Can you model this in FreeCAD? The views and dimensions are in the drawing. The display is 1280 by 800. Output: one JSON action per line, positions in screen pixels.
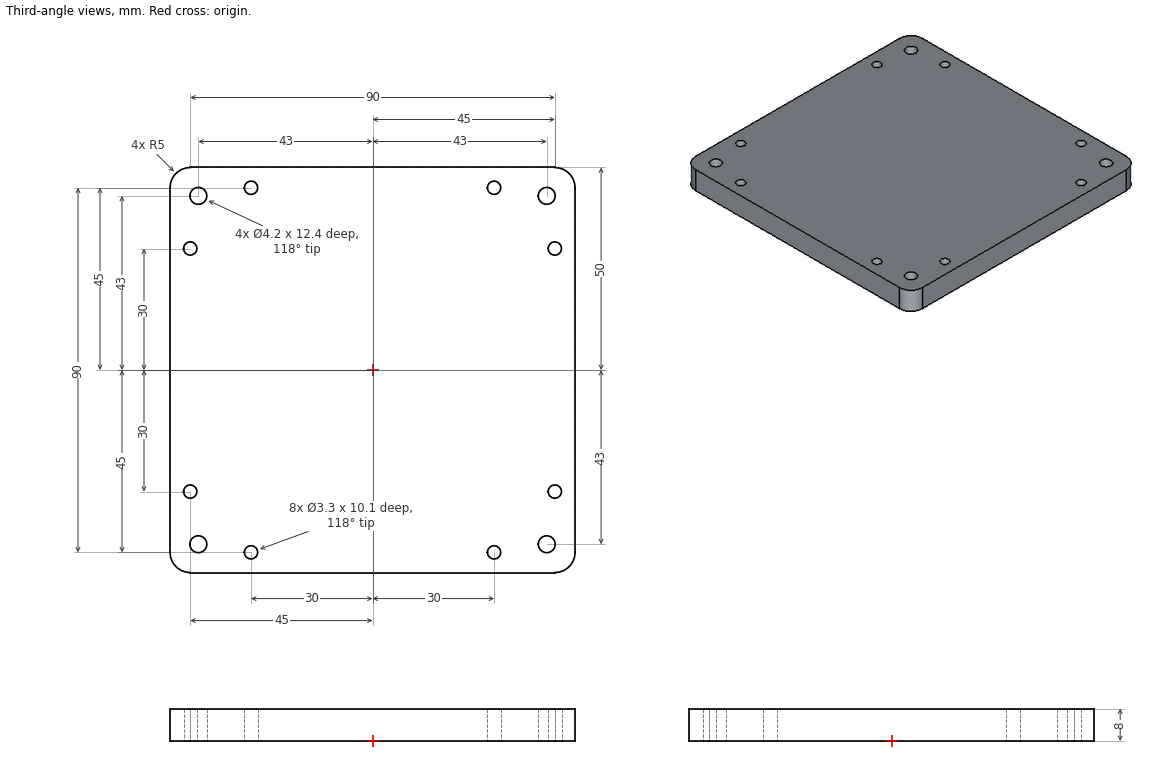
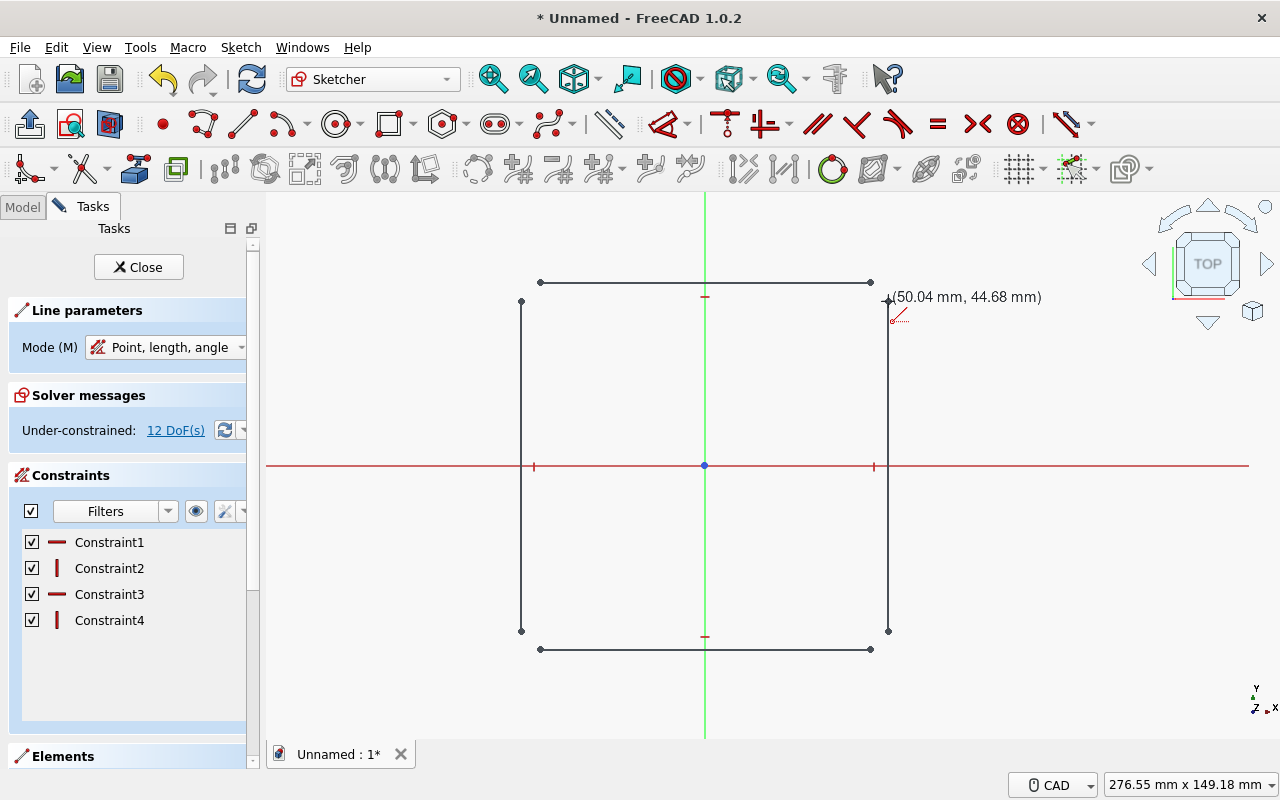
{"action": "key", "text": "g 3 a"}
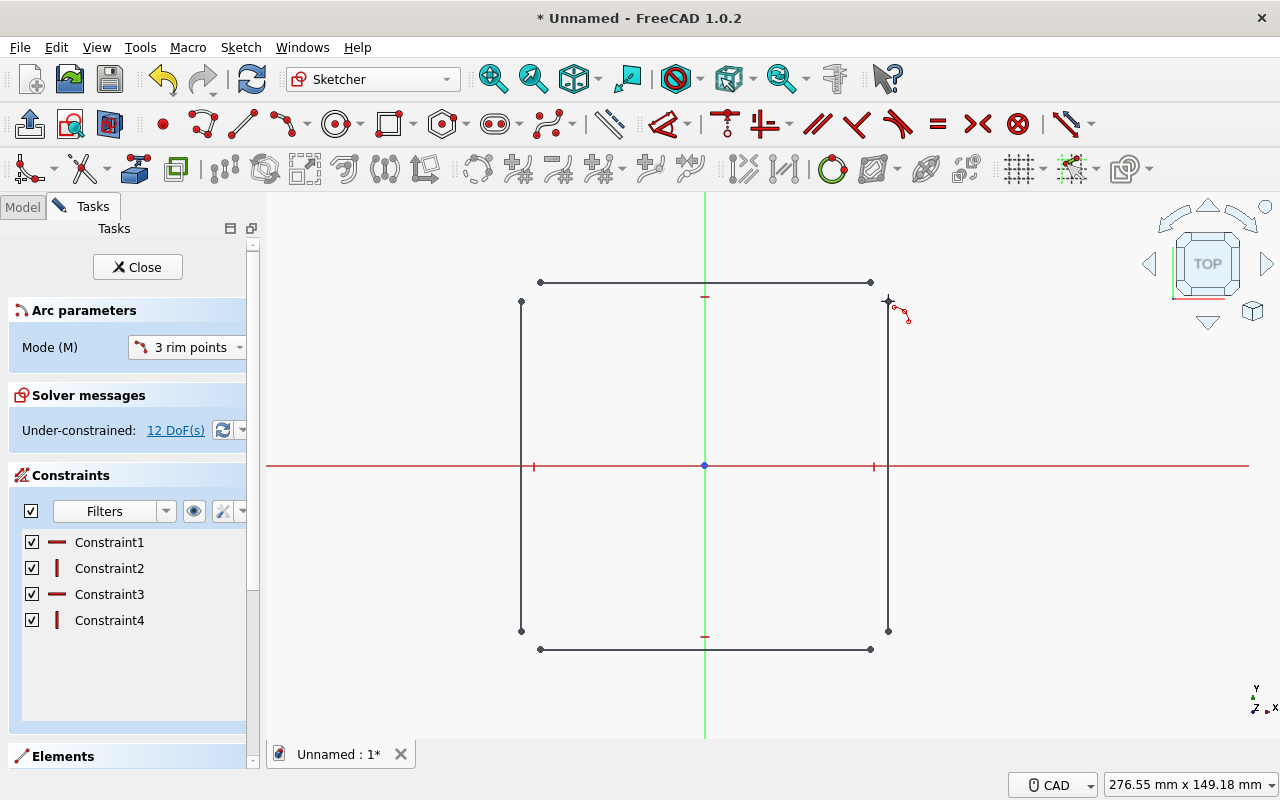
{"action": "left_click", "coordinate": [540, 283]}
{"action": "left_click", "coordinate": [521, 302]}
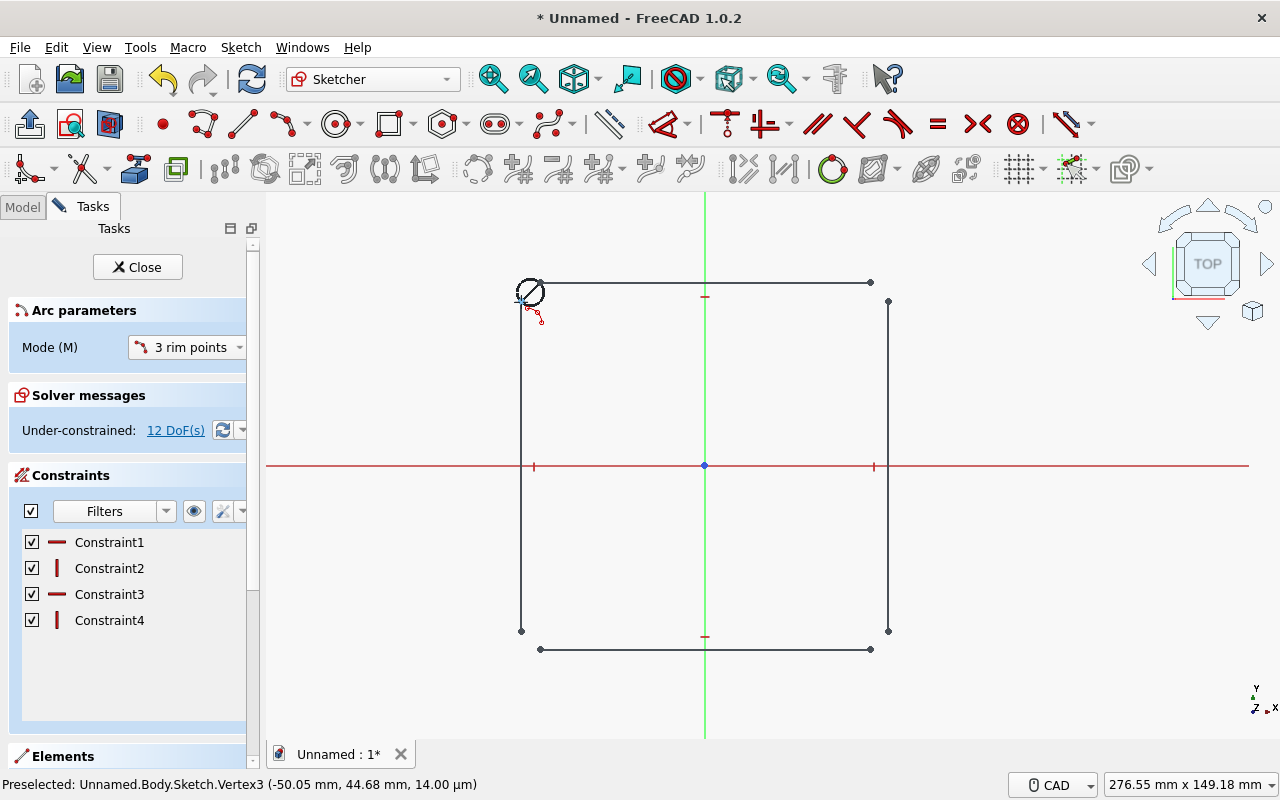
{"action": "scroll", "coordinate": [527, 288], "scroll_direction": "up", "scroll_amount": 6}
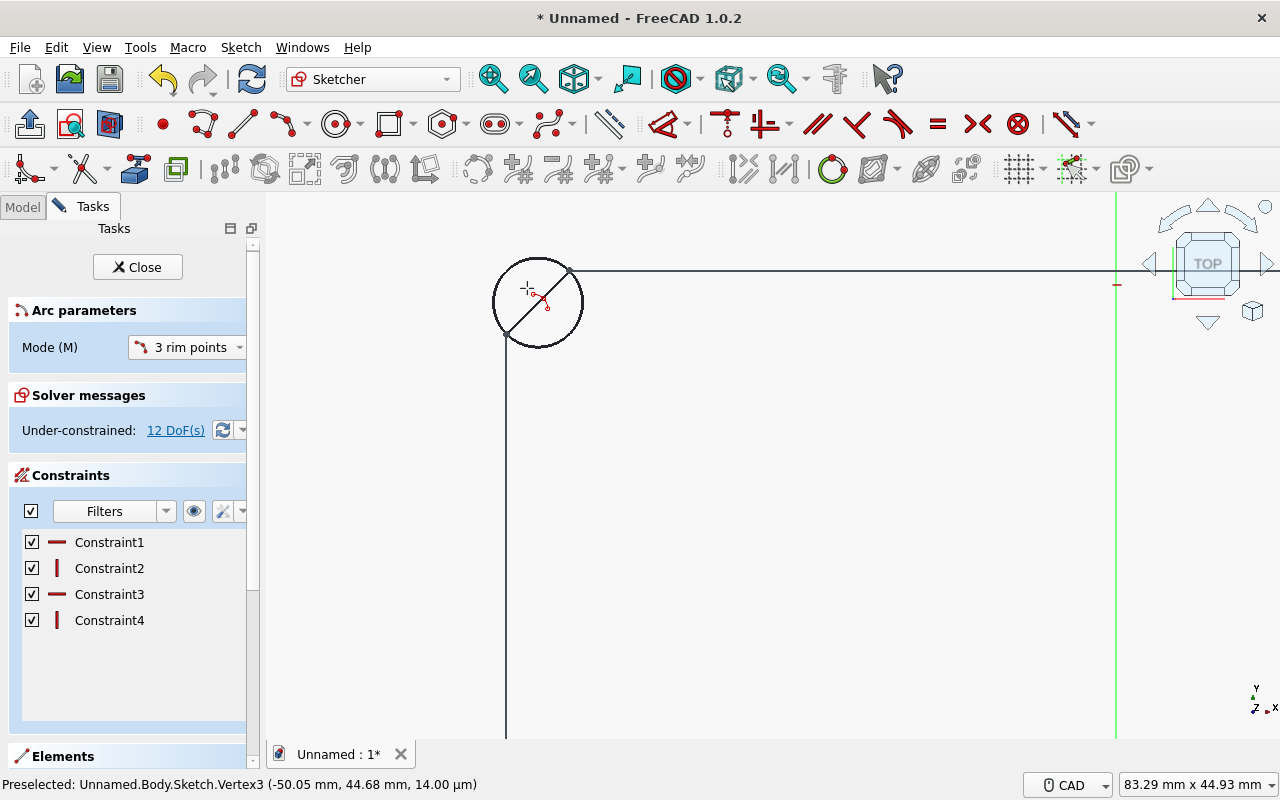
{"action": "left_click", "coordinate": [525, 287]}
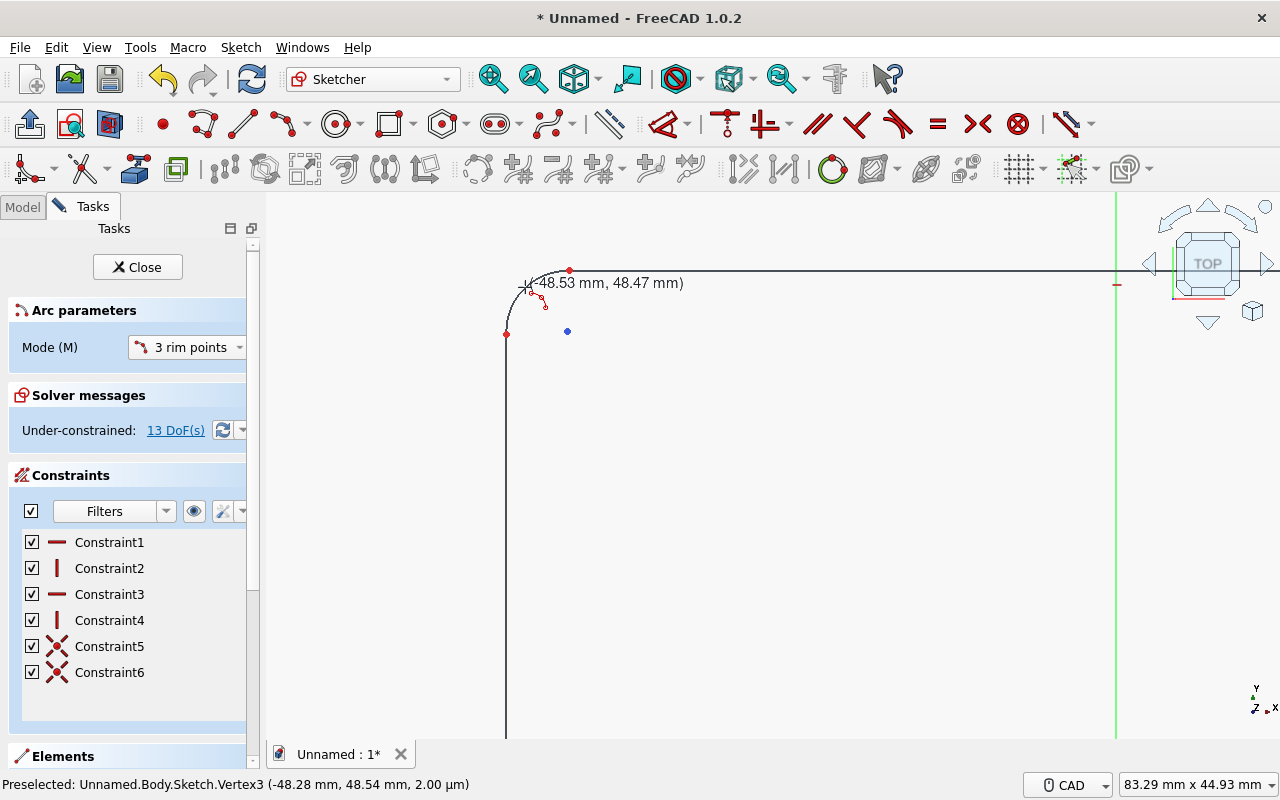
{"action": "scroll", "coordinate": [527, 288], "scroll_direction": "down", "scroll_amount": 6}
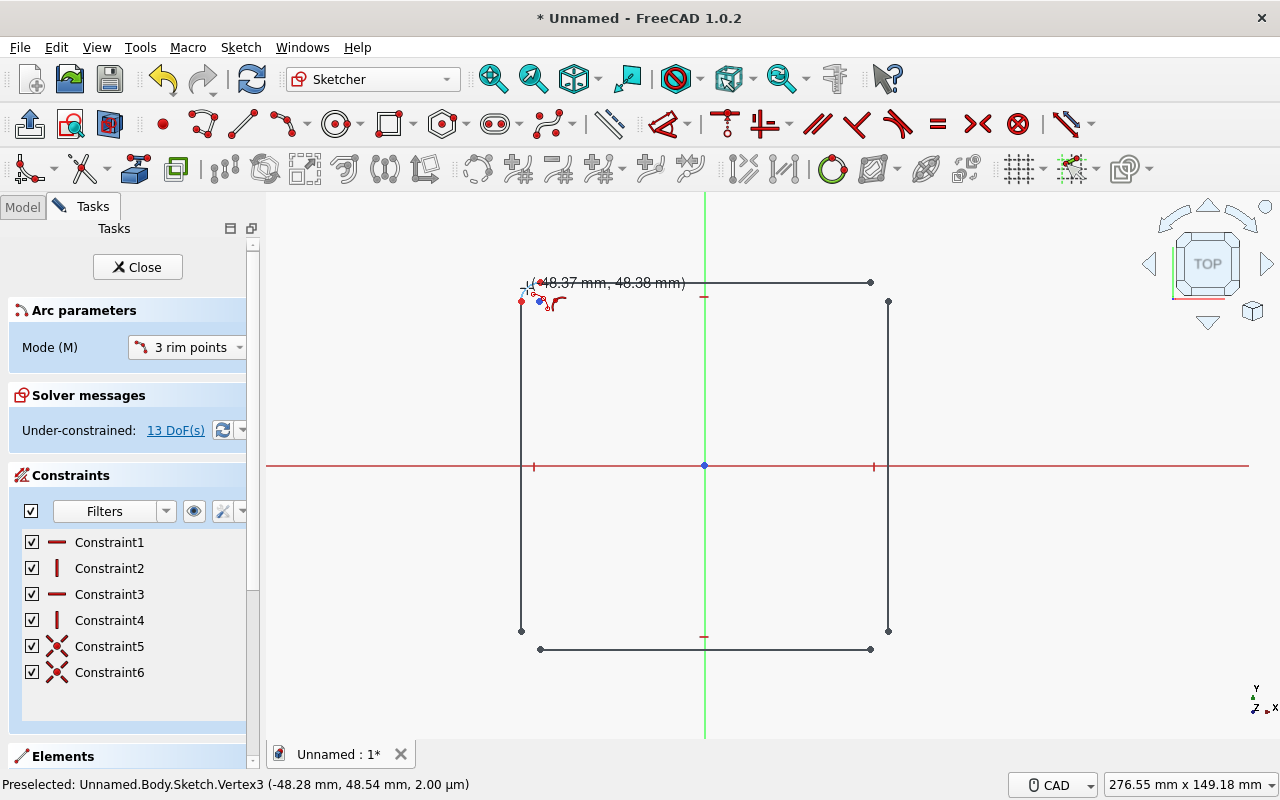
{"action": "left_click", "coordinate": [521, 632]}
{"action": "left_click", "coordinate": [540, 650]}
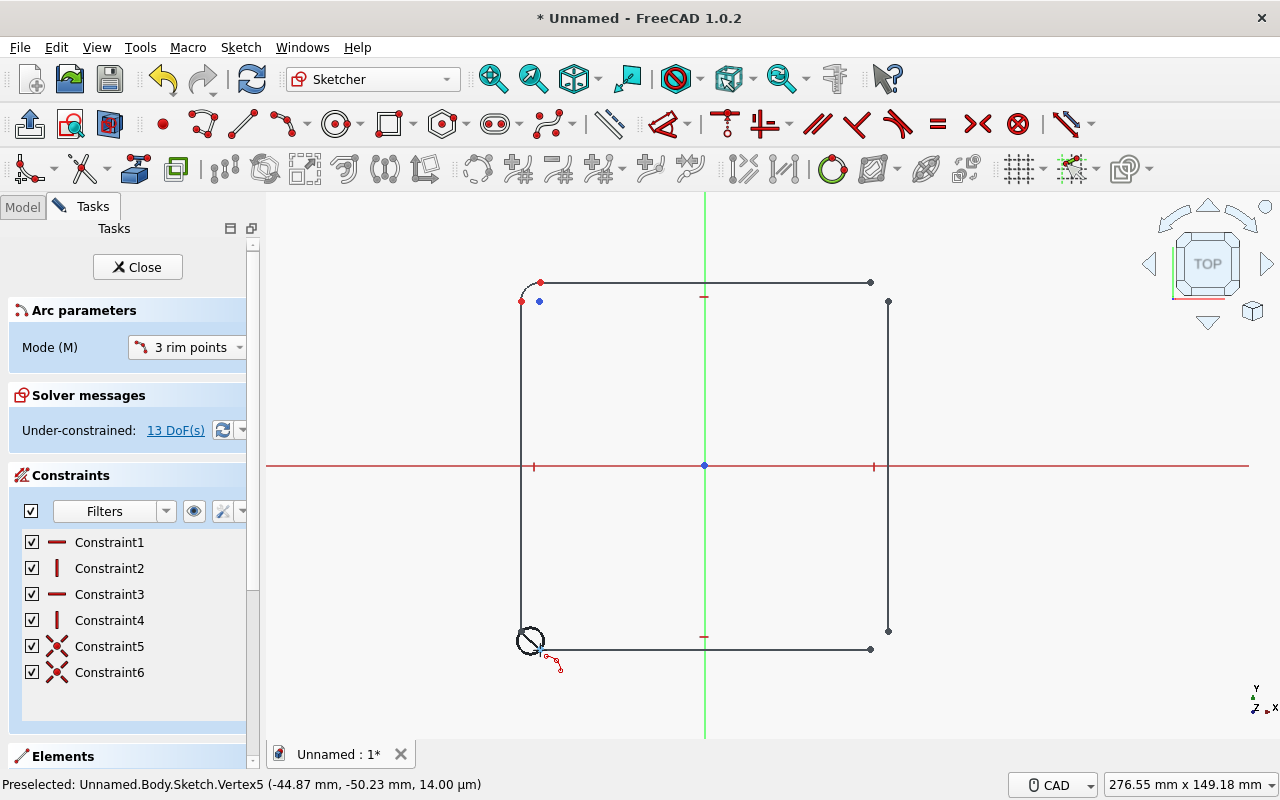
{"action": "scroll", "coordinate": [527, 644], "scroll_direction": "up", "scroll_amount": 6}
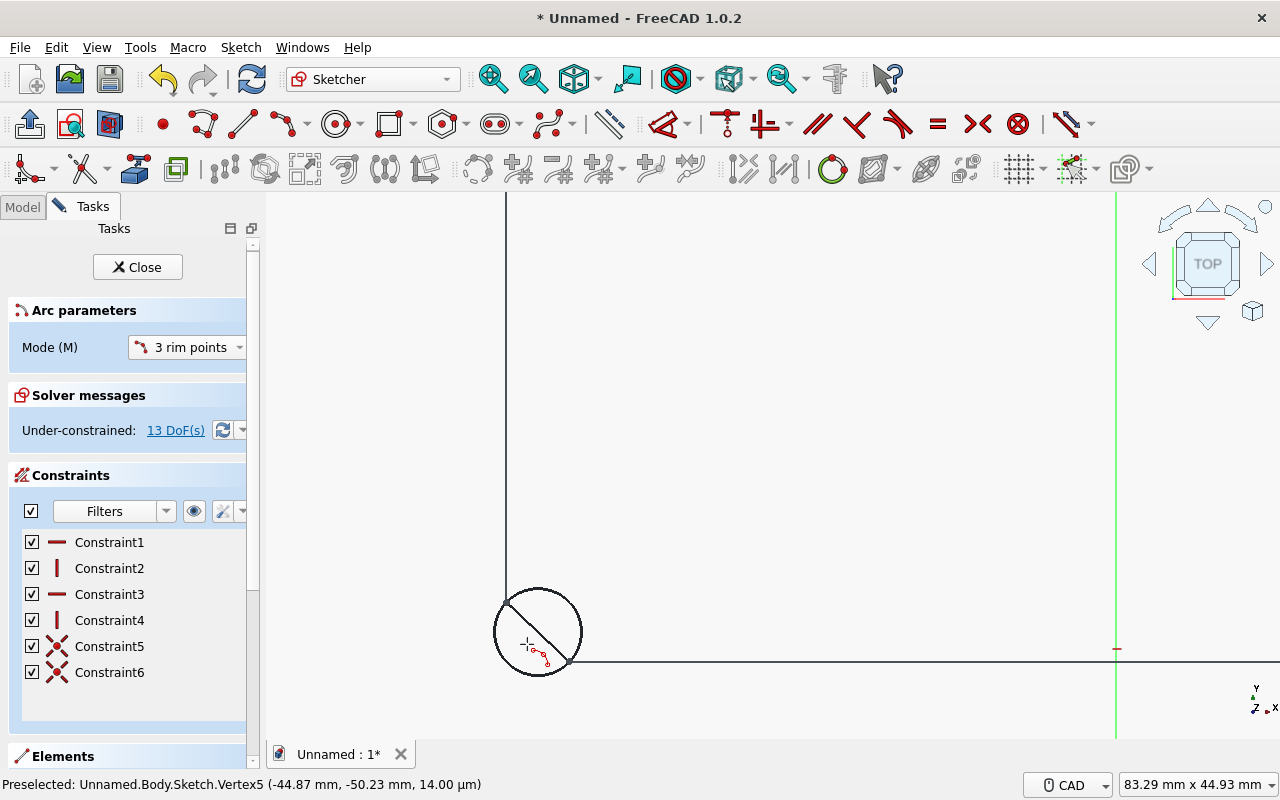
{"action": "left_click", "coordinate": [525, 641]}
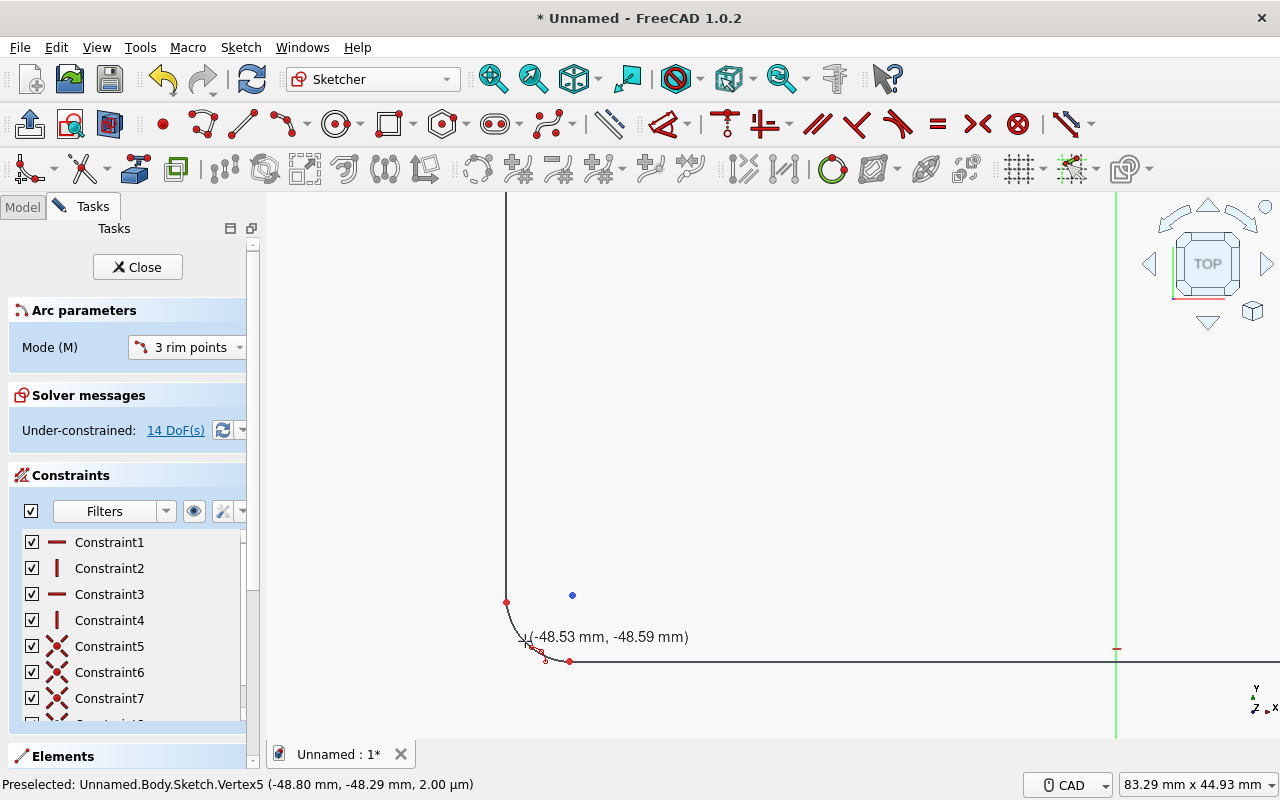
{"action": "scroll", "coordinate": [527, 644], "scroll_direction": "down", "scroll_amount": 6}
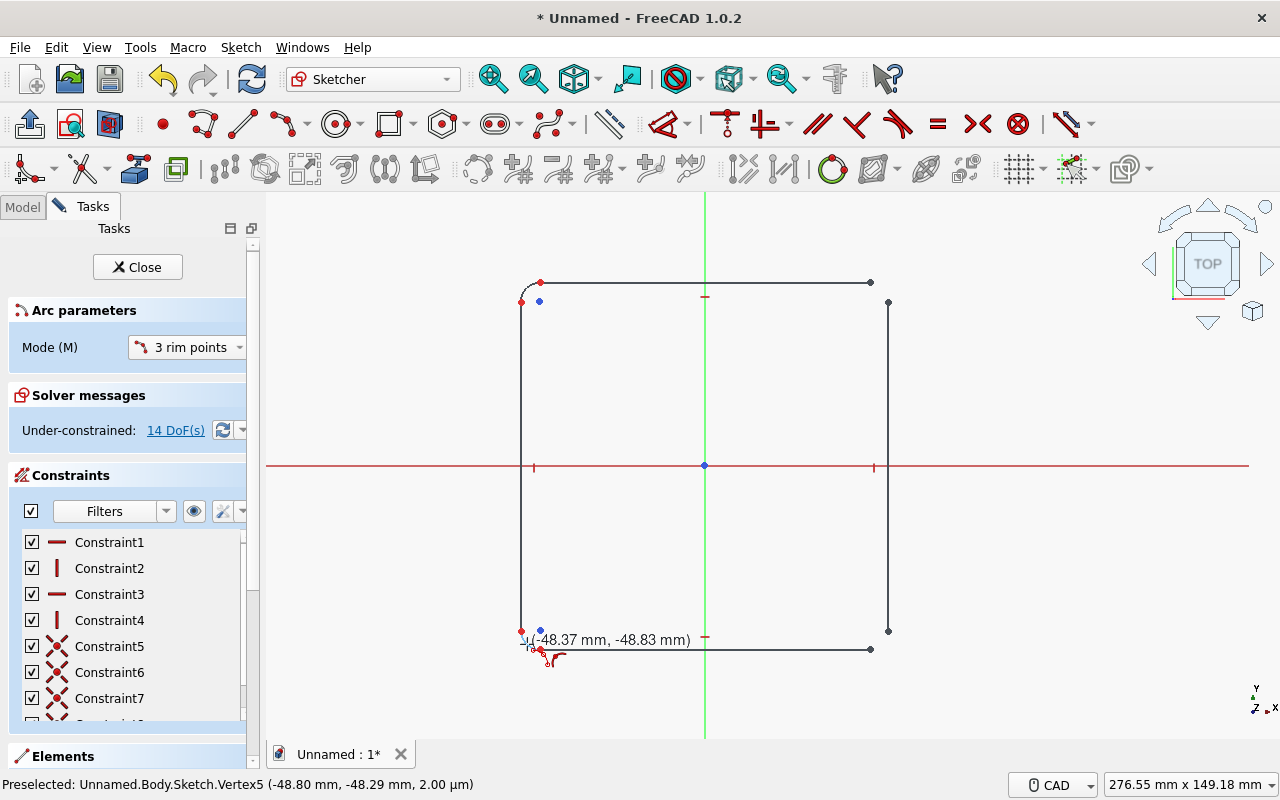
{"action": "left_click", "coordinate": [870, 650]}
{"action": "left_click", "coordinate": [888, 632]}